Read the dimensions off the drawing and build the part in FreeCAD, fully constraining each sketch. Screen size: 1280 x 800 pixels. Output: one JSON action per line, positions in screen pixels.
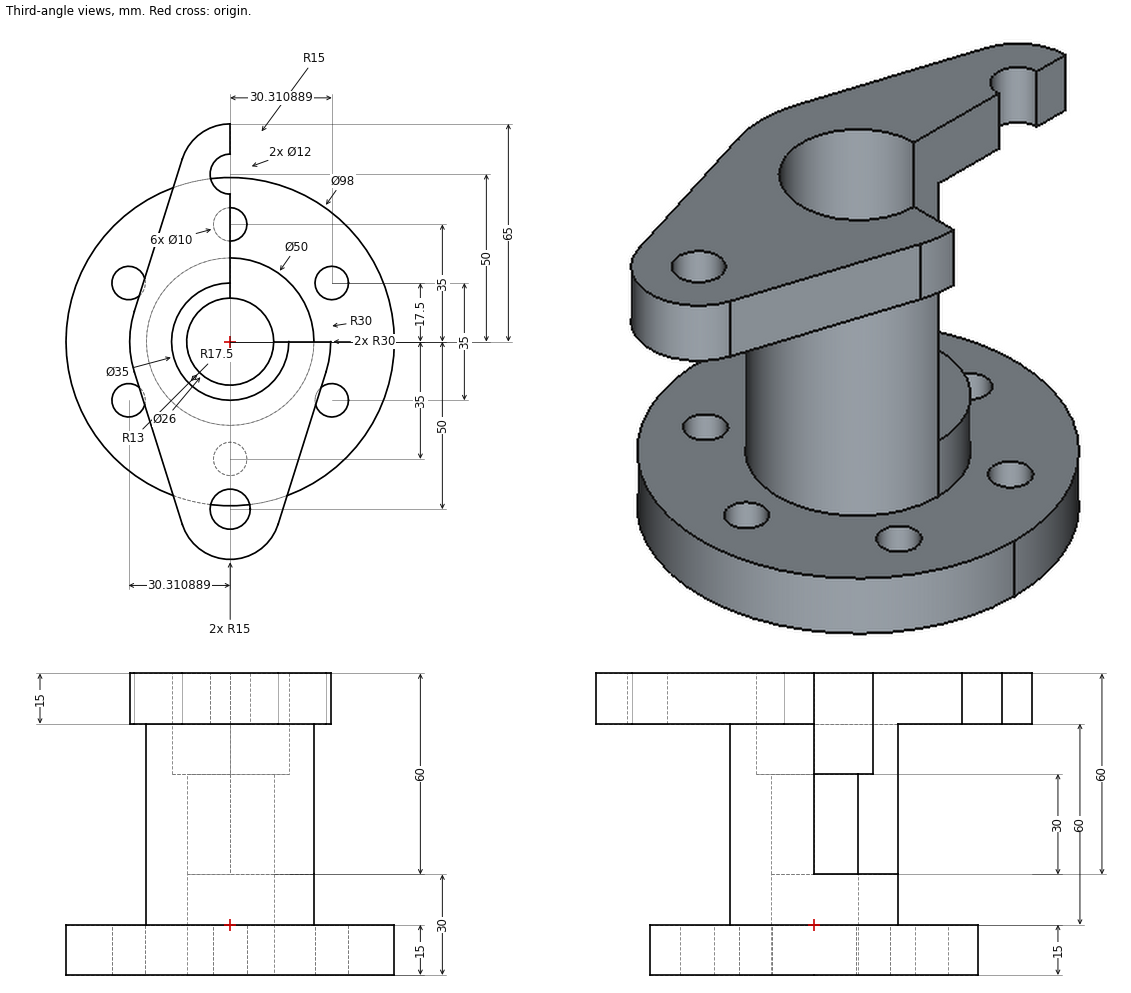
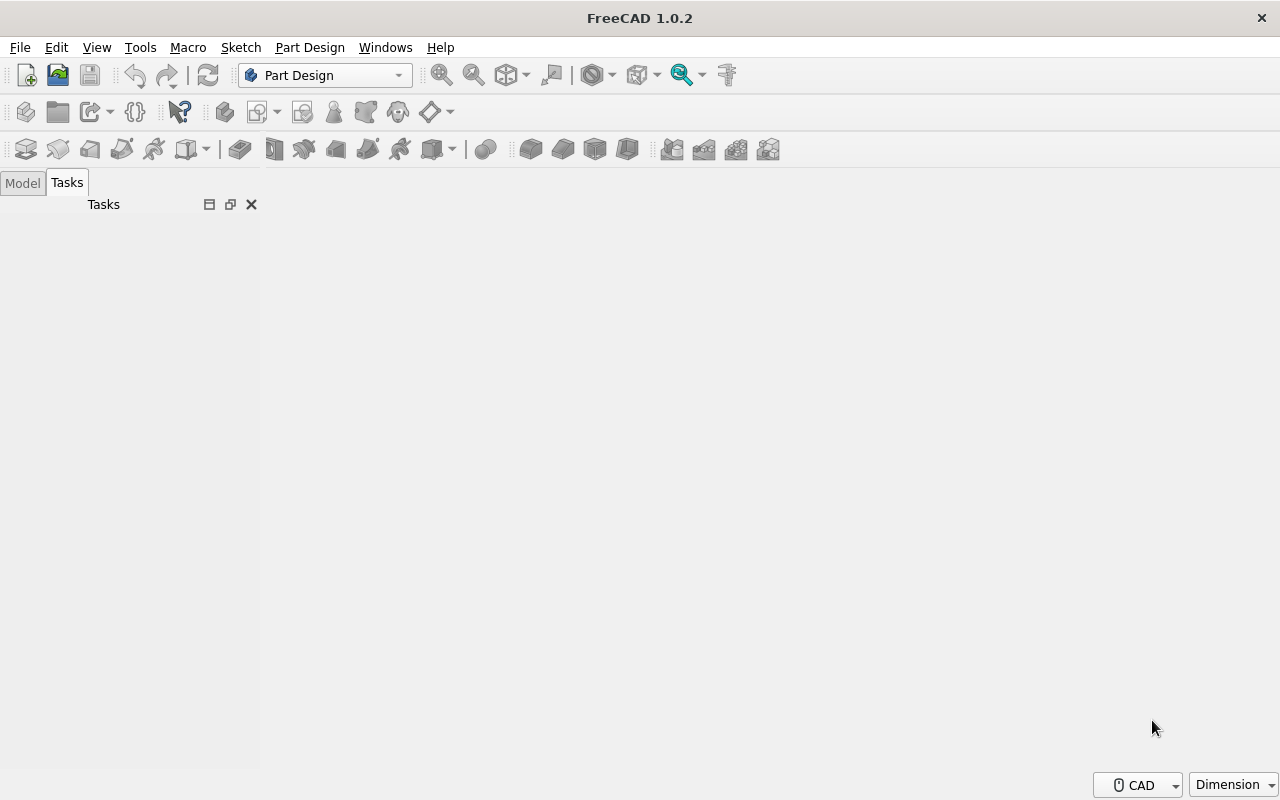
{"action": "left_click", "coordinate": [616, 112]}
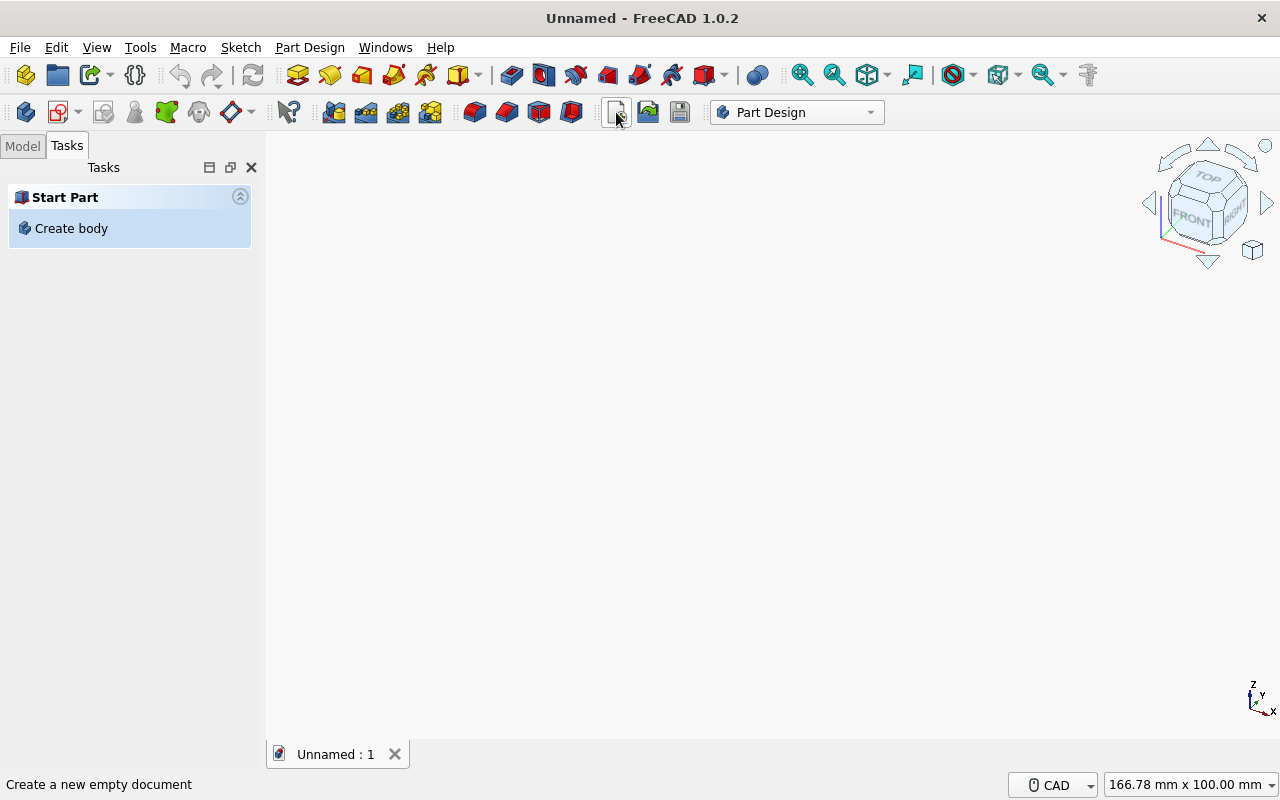
{"action": "left_click", "coordinate": [58, 112]}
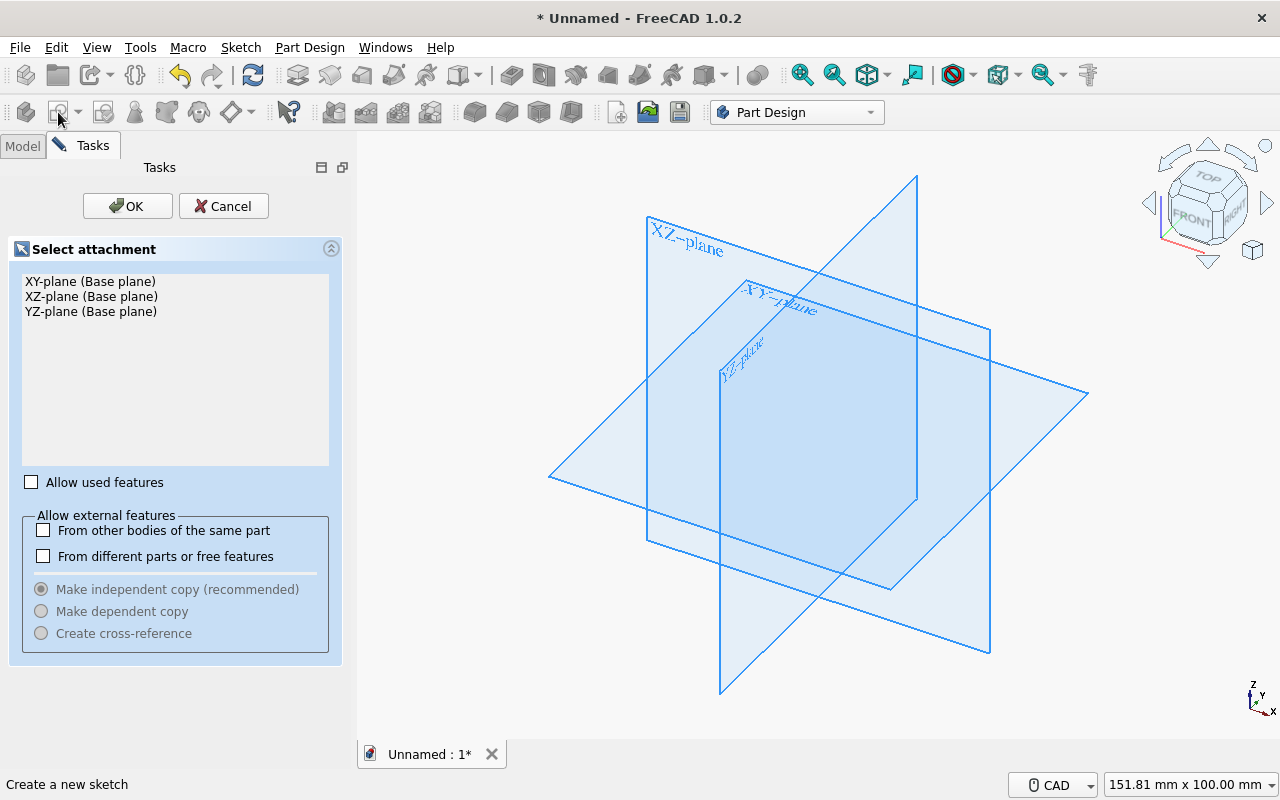
{"action": "left_click", "coordinate": [82, 282]}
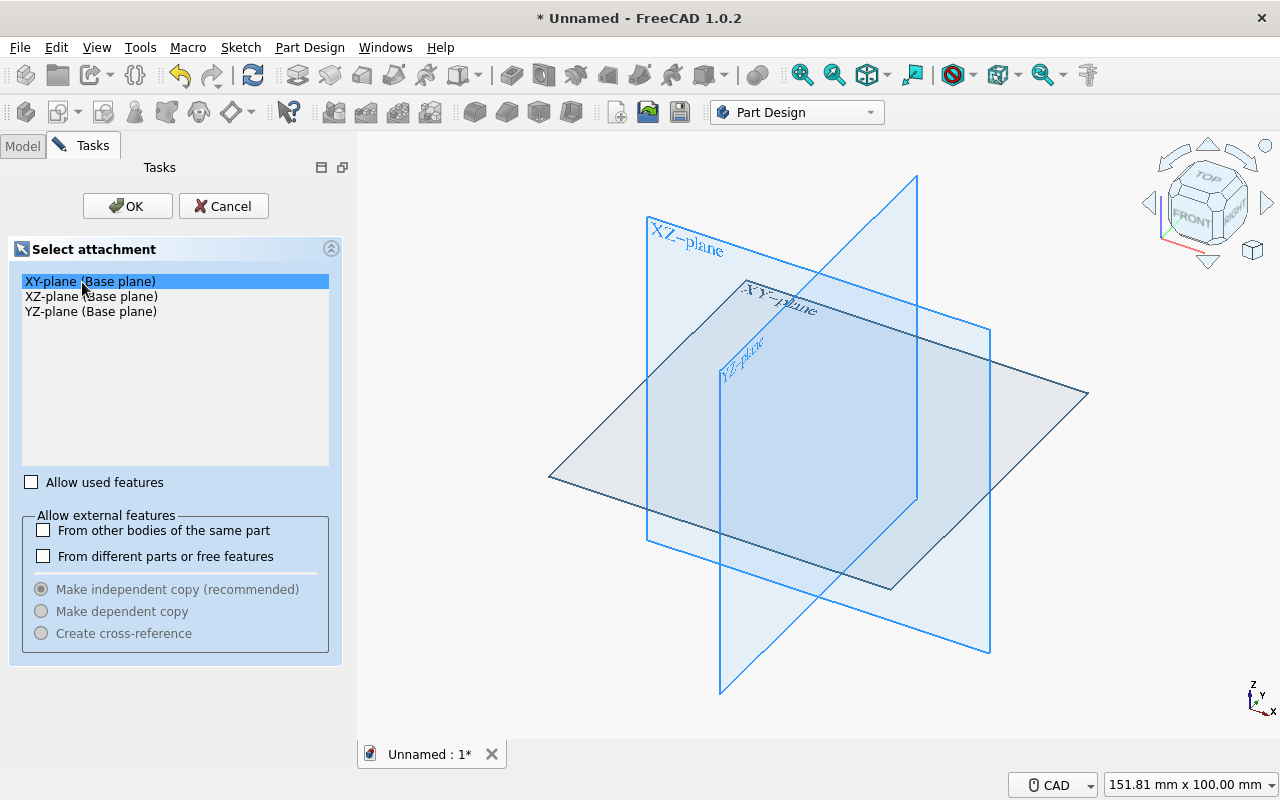
{"action": "left_click", "coordinate": [128, 206]}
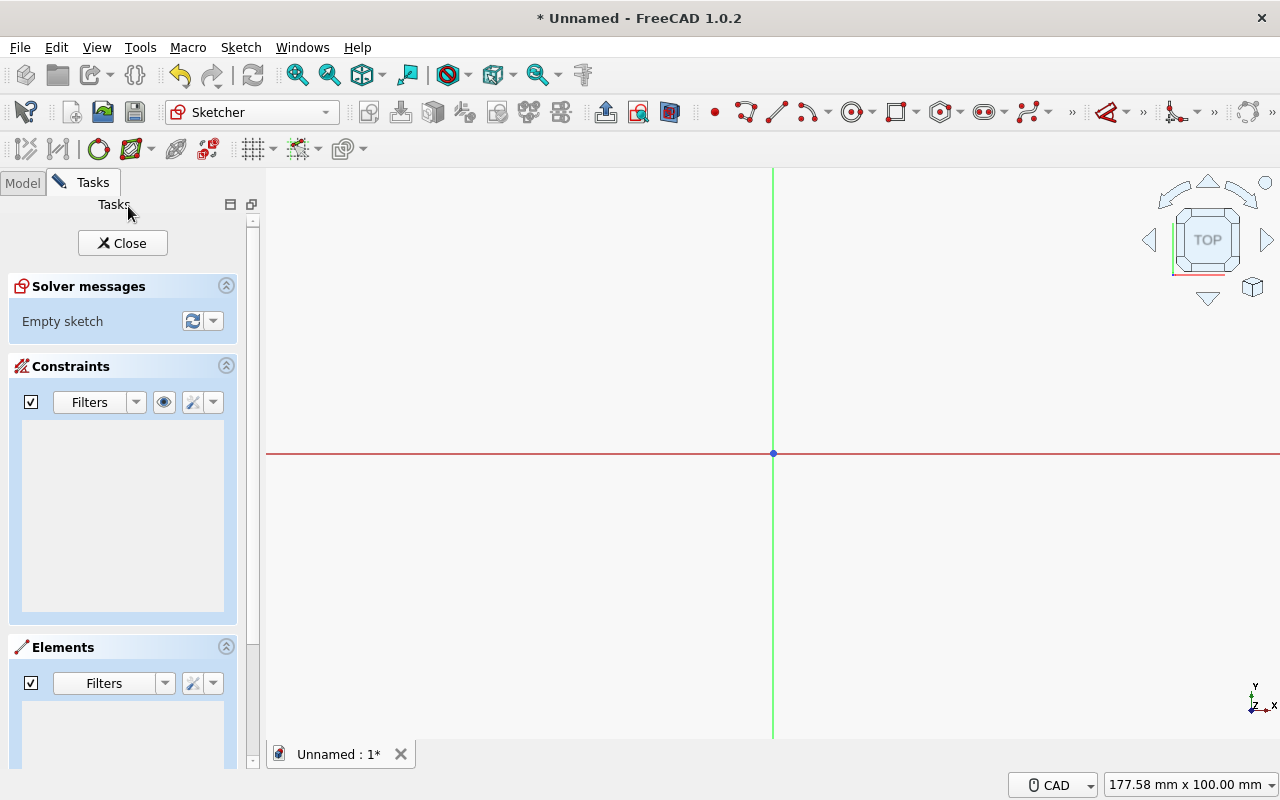
{"action": "scroll", "coordinate": [565, 453], "scroll_direction": "down", "scroll_amount": 2}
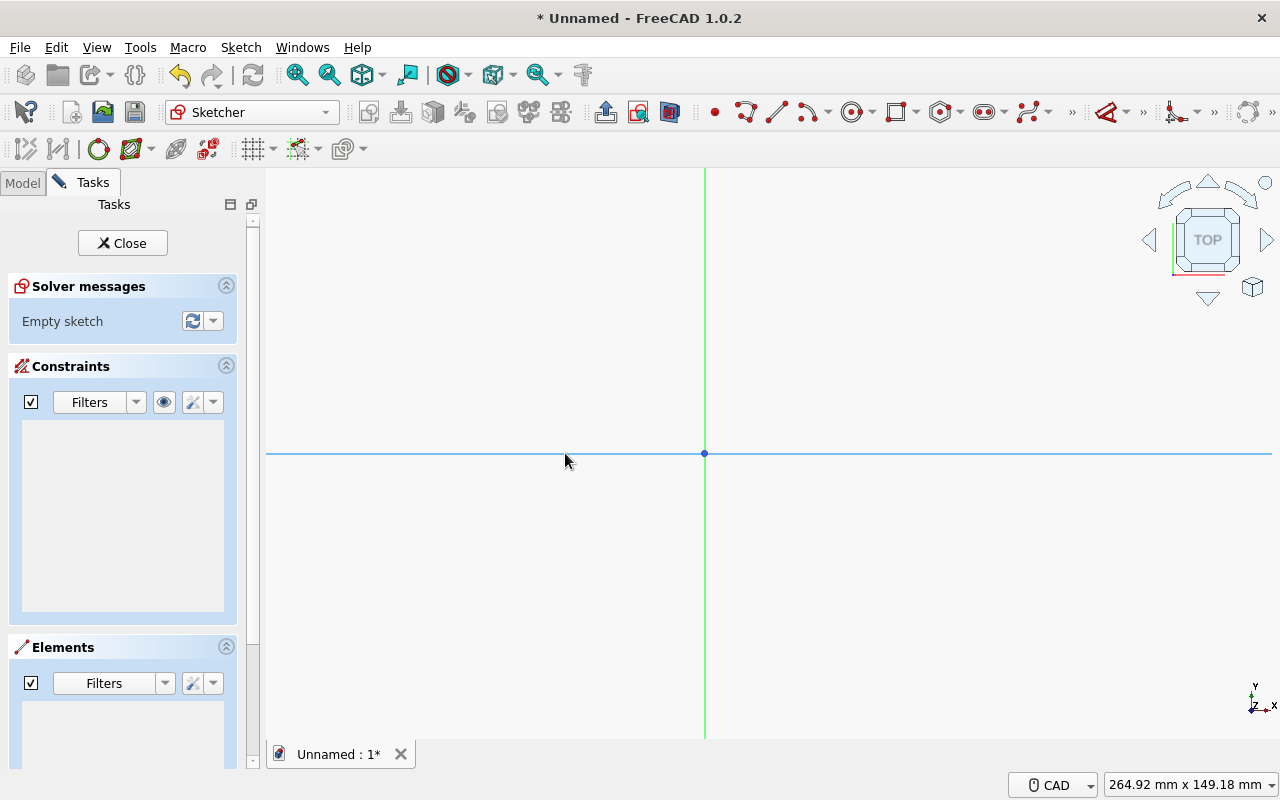
{"action": "left_click", "coordinate": [852, 112]}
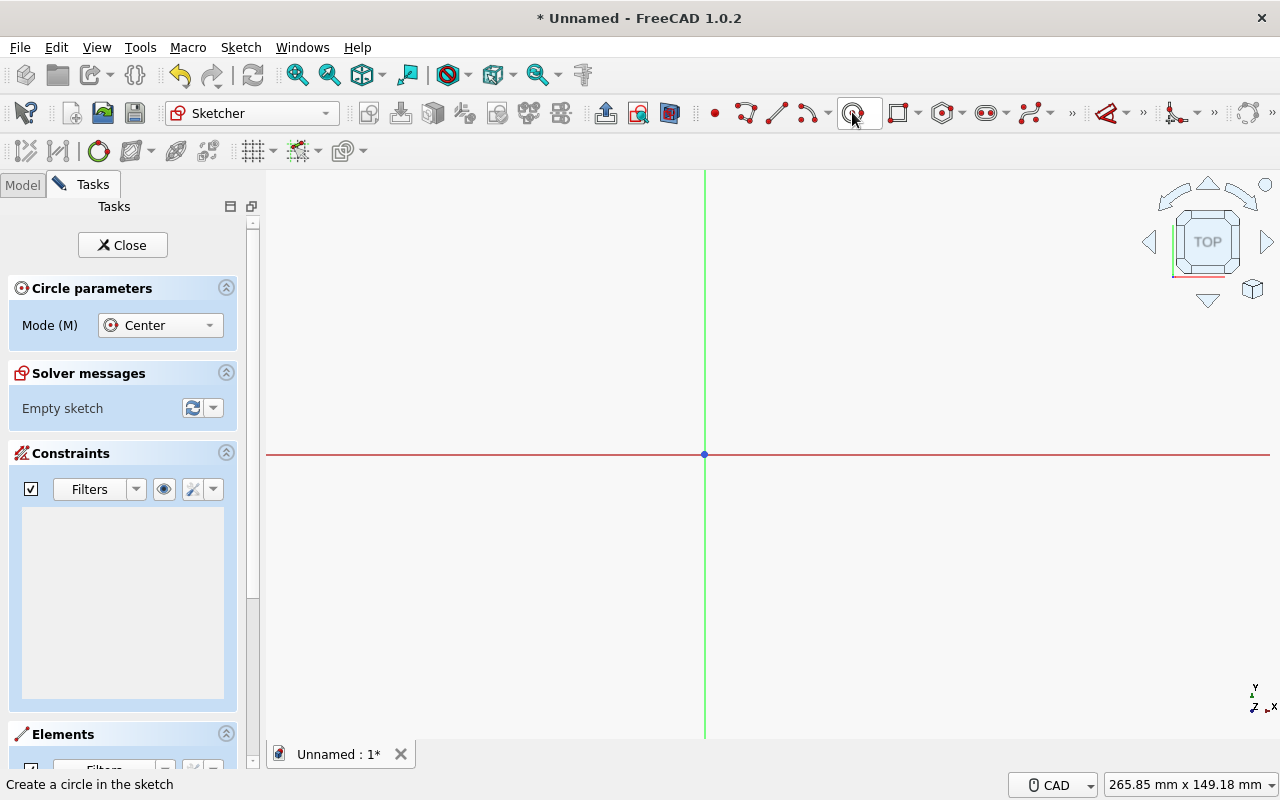
{"action": "left_click", "coordinate": [705, 454]}
{"action": "left_click", "coordinate": [837, 322]}
{"action": "key", "text": "Escape"}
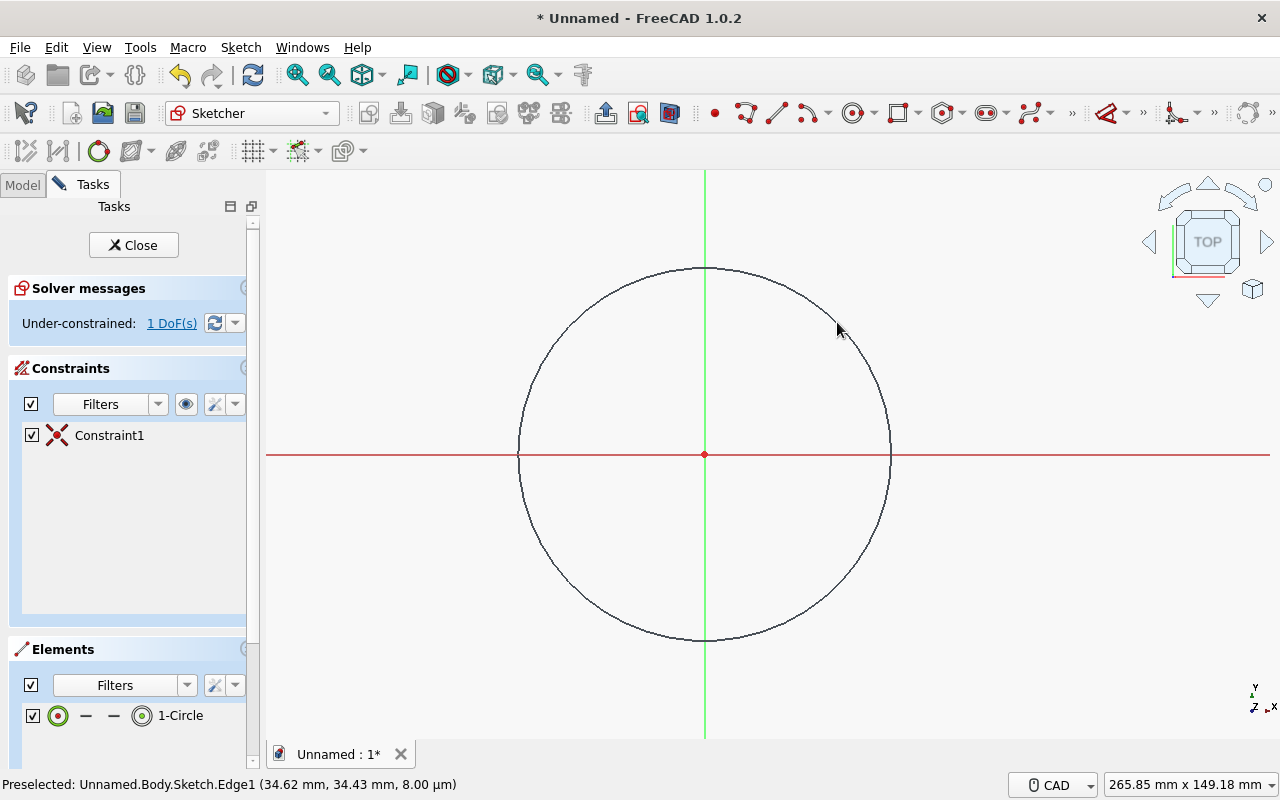
{"action": "left_click", "coordinate": [836, 322]}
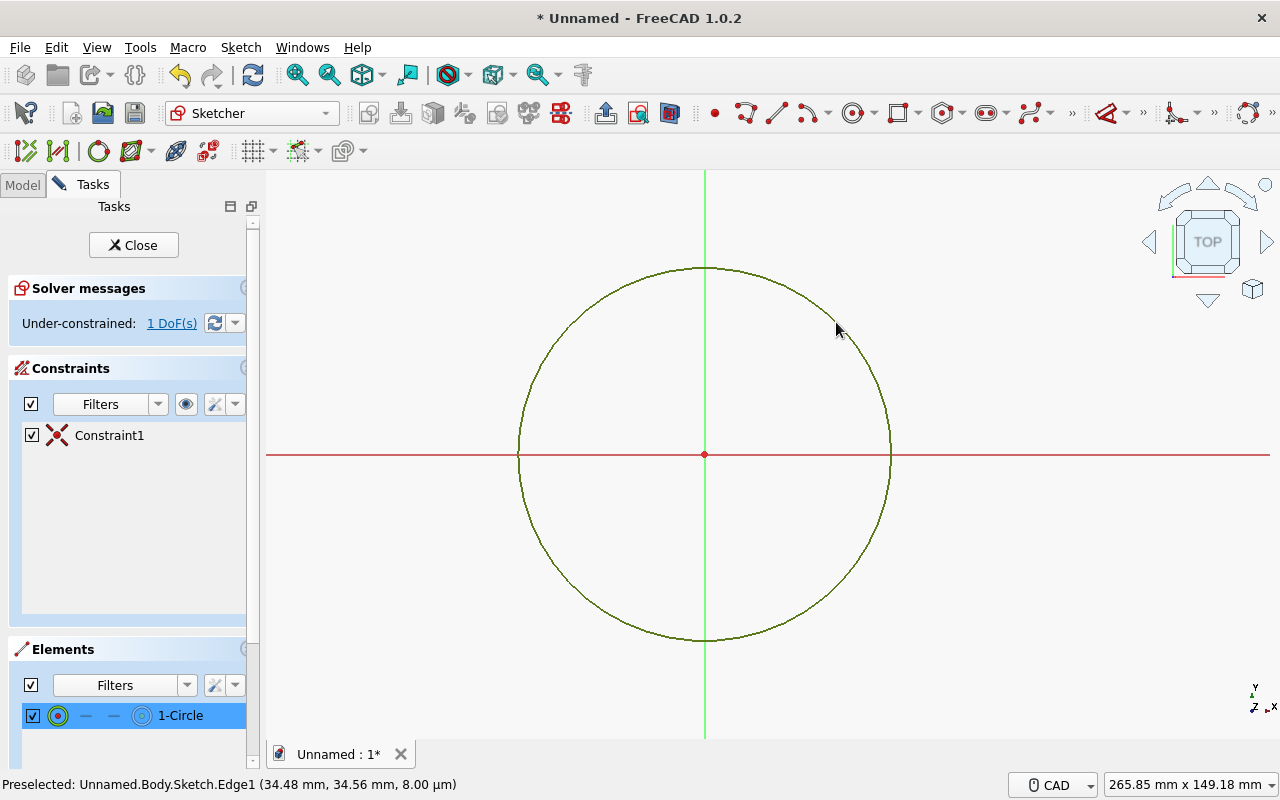
{"action": "key", "text": "k o"}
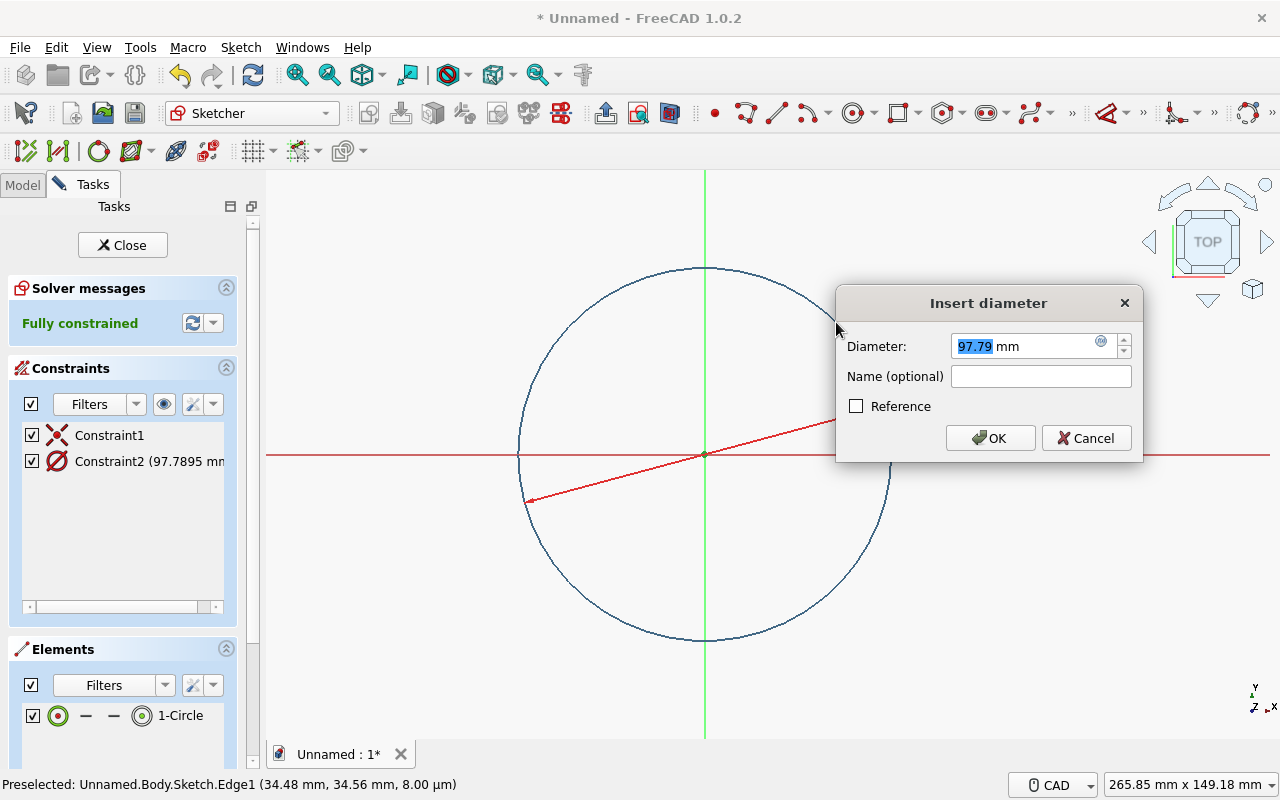
{"action": "type", "text": "98"}
{"action": "key", "text": "Return"}